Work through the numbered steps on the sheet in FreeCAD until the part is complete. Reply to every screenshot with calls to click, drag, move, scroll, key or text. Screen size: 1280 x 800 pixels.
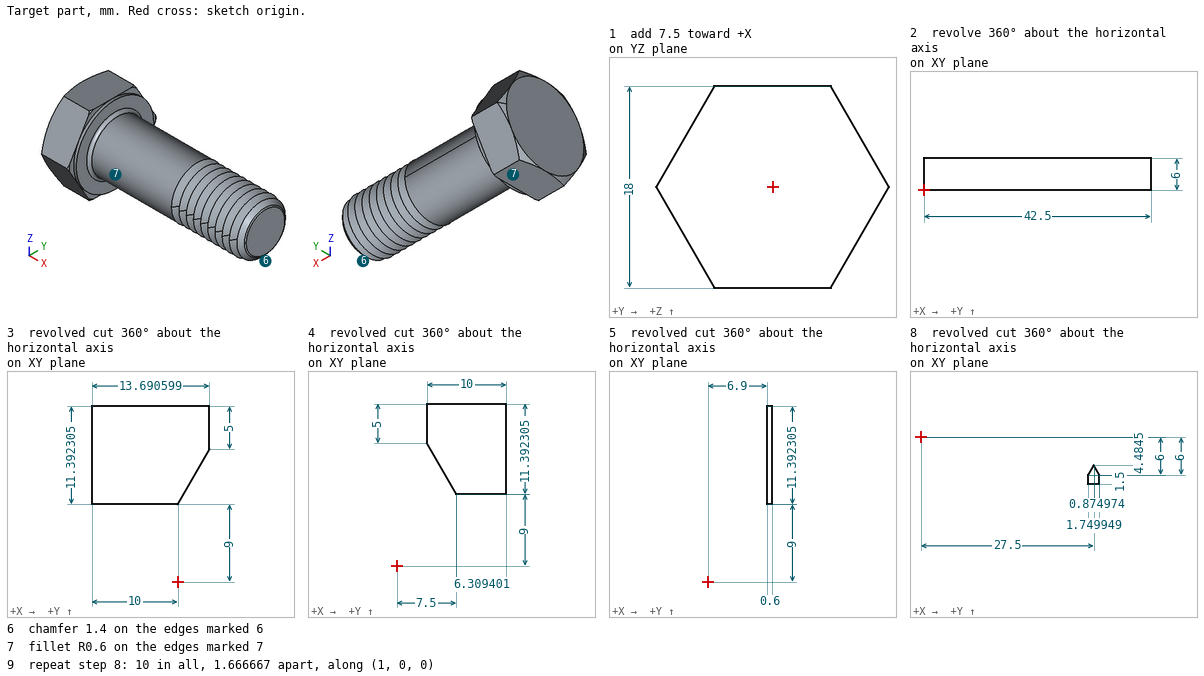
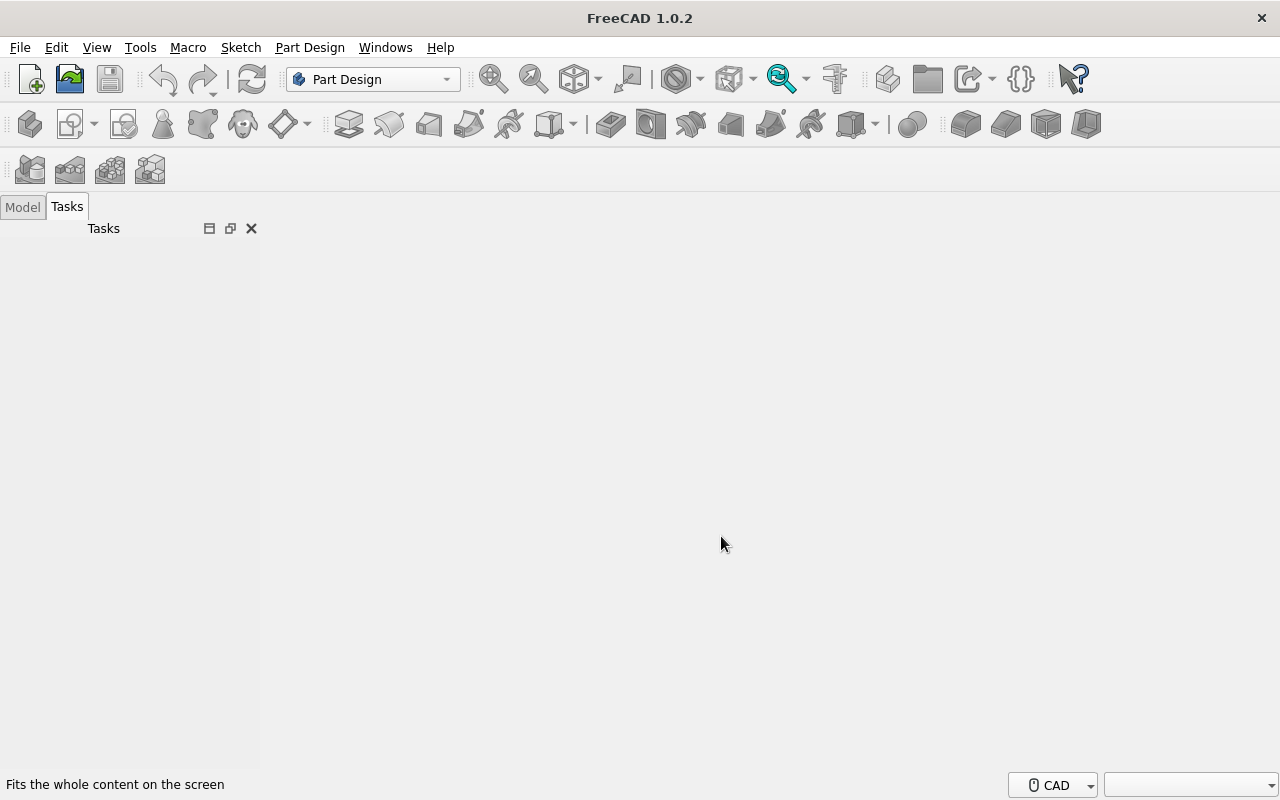
click(30, 80)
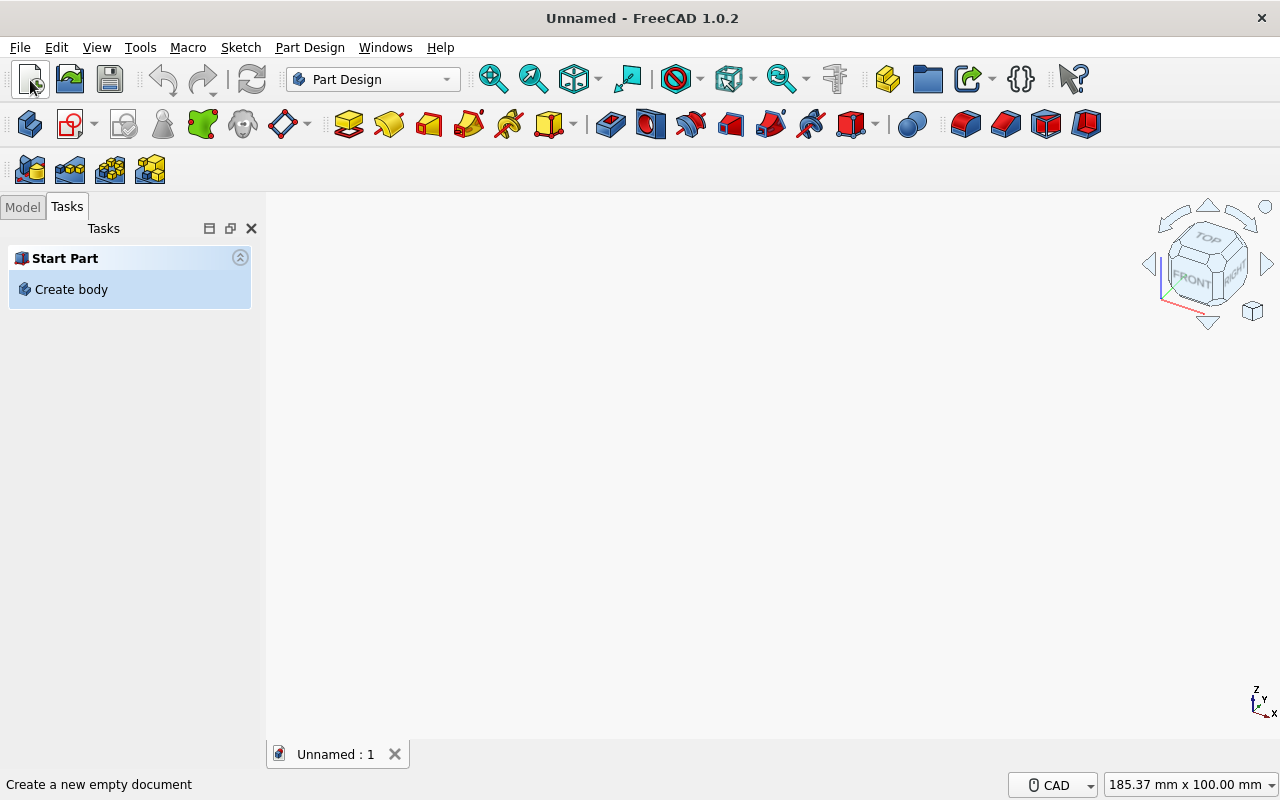
click(70, 124)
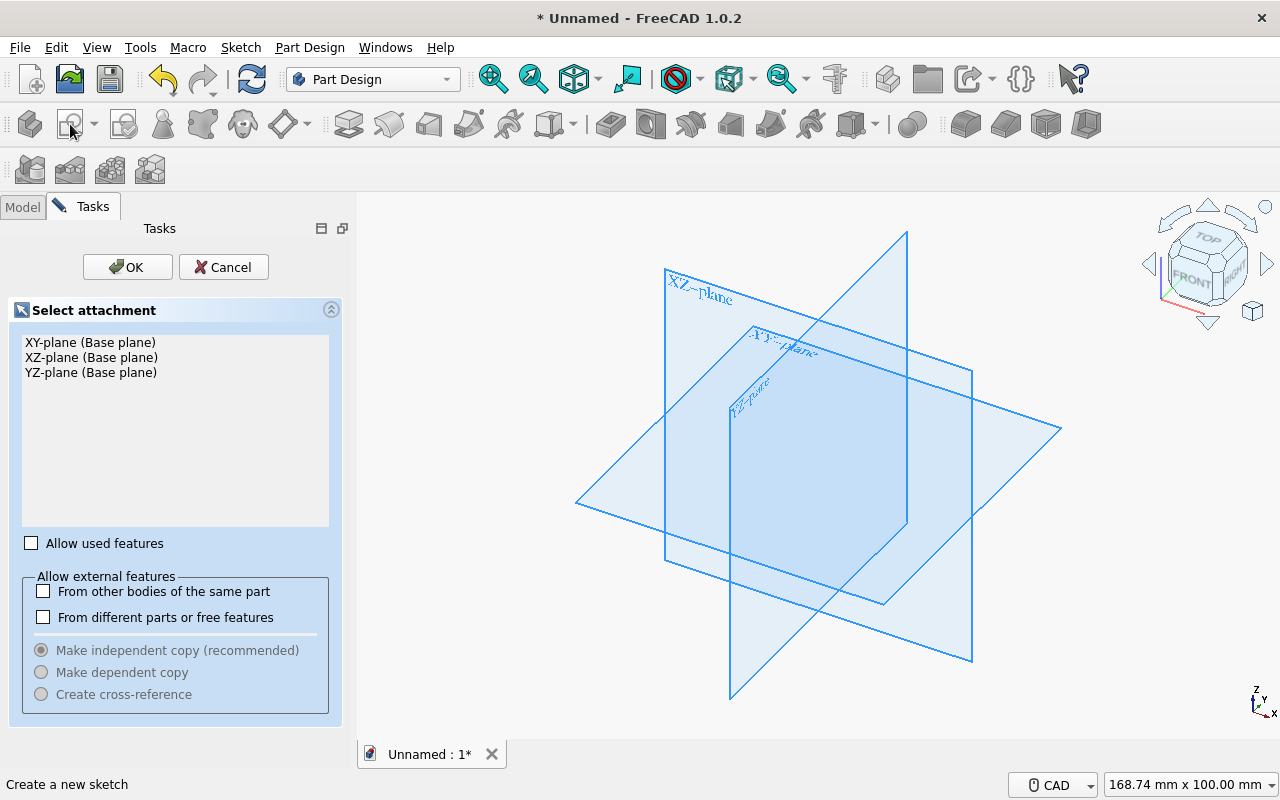
click(82, 372)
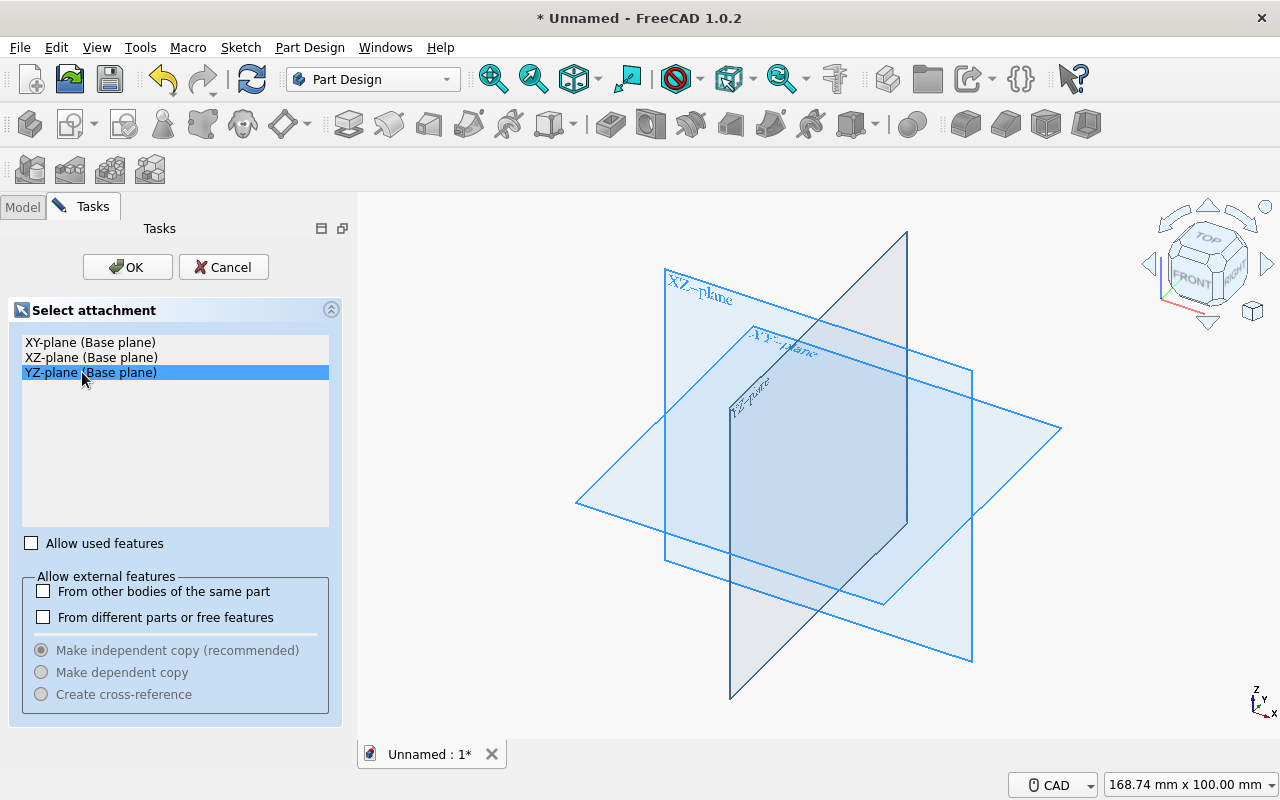
click(128, 267)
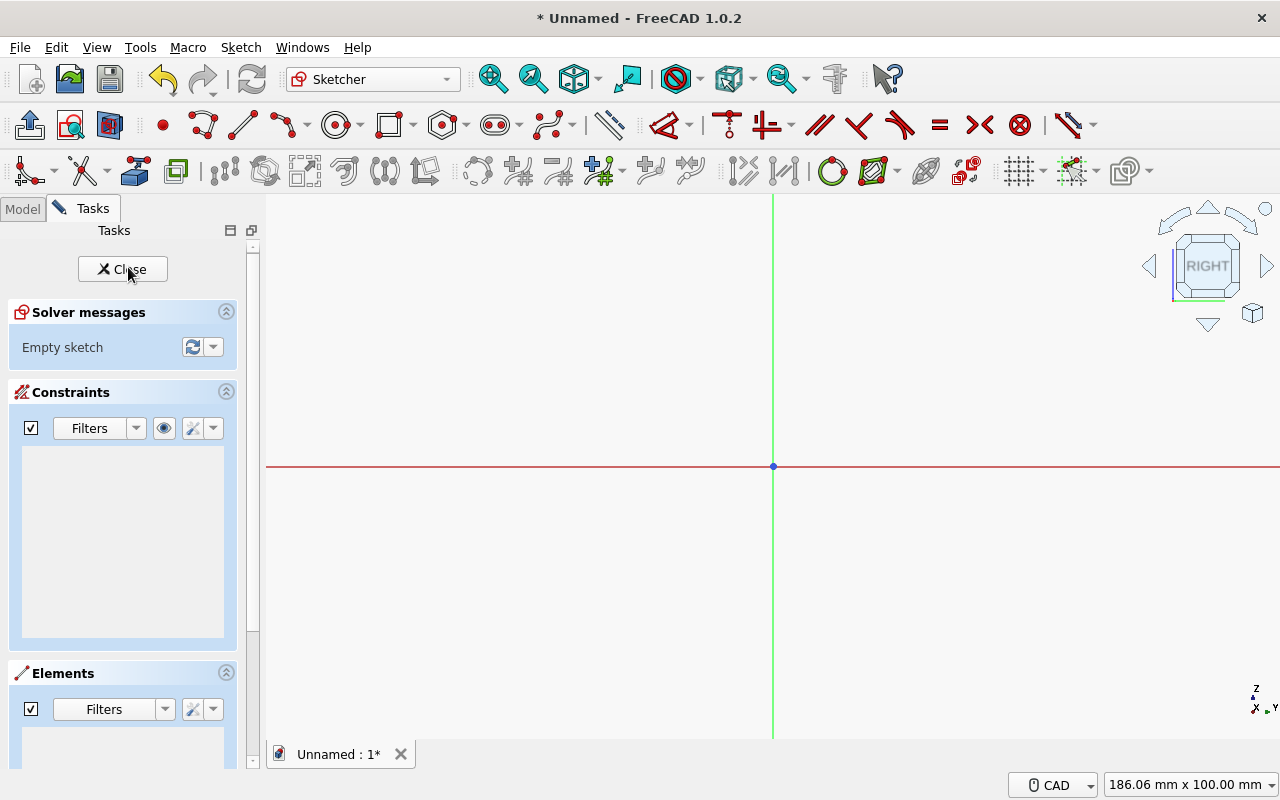
scroll(803, 466, up, 6)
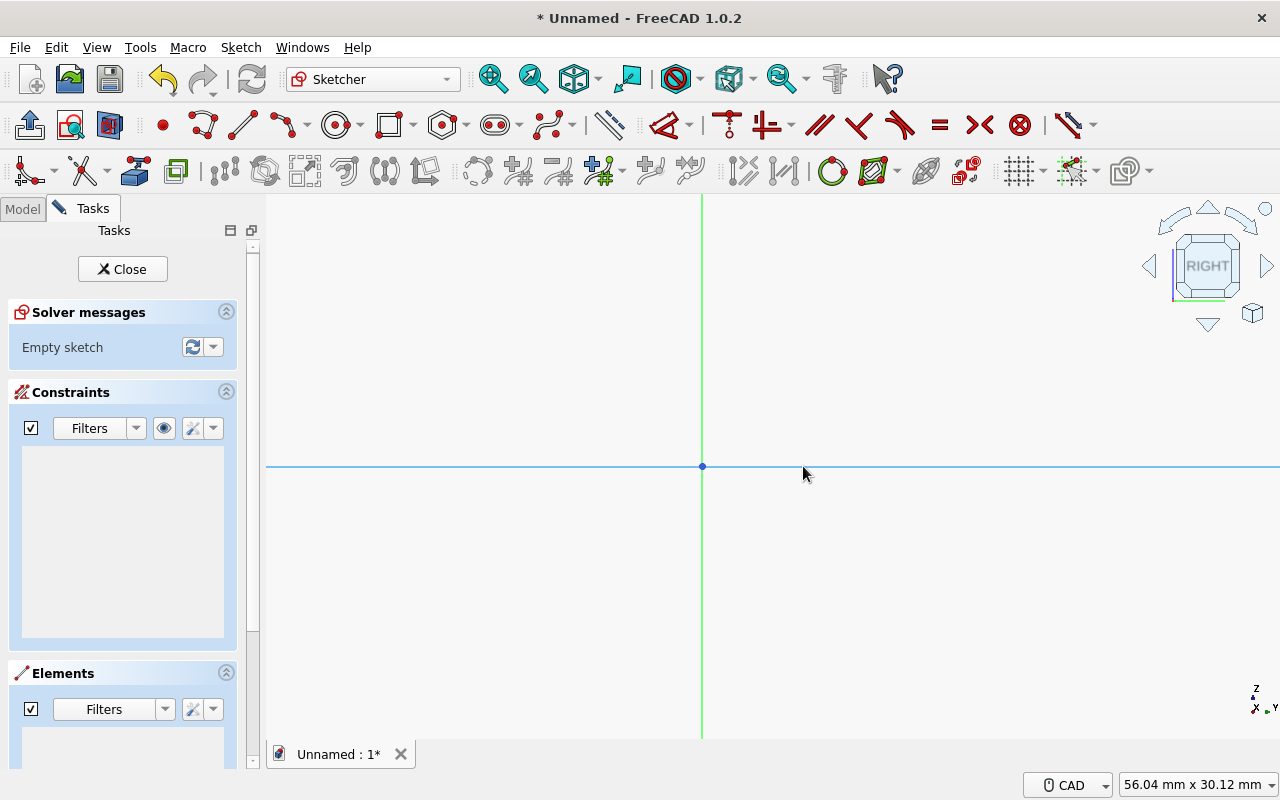
click(442, 126)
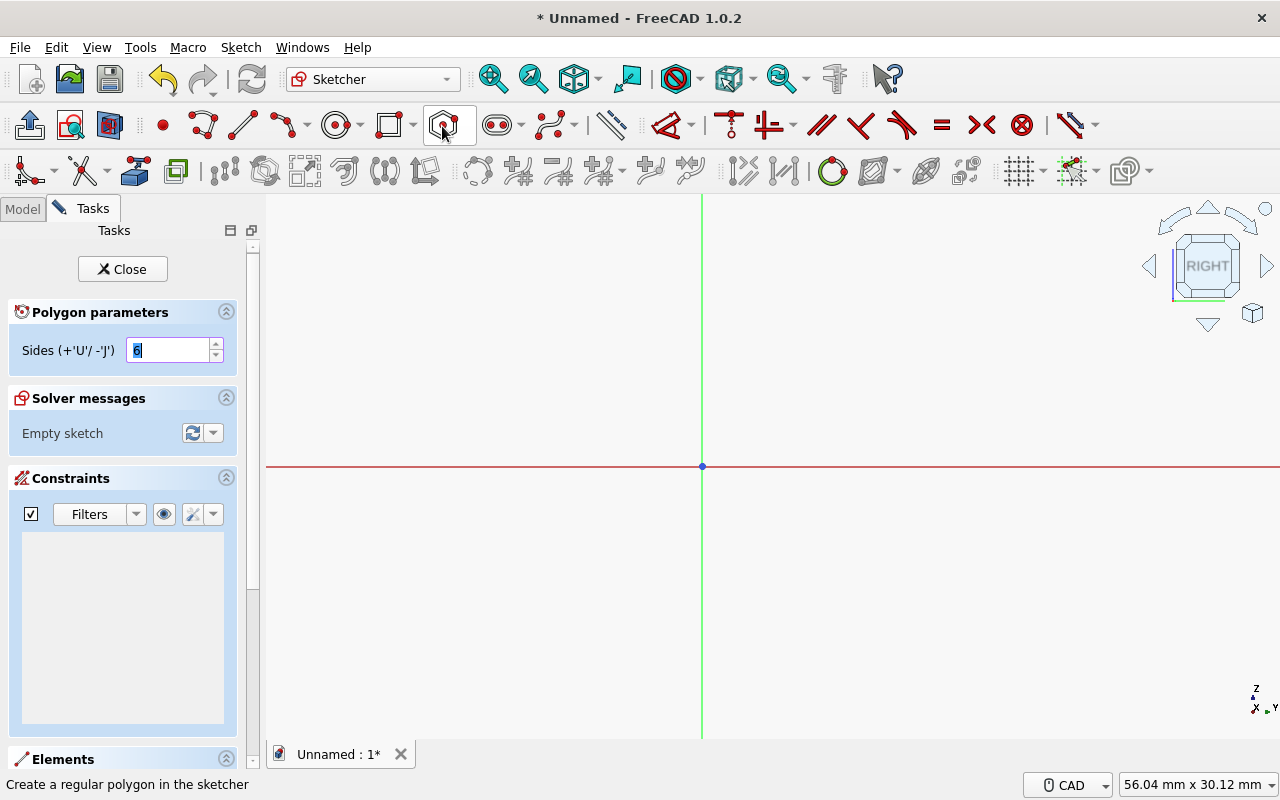
click(702, 466)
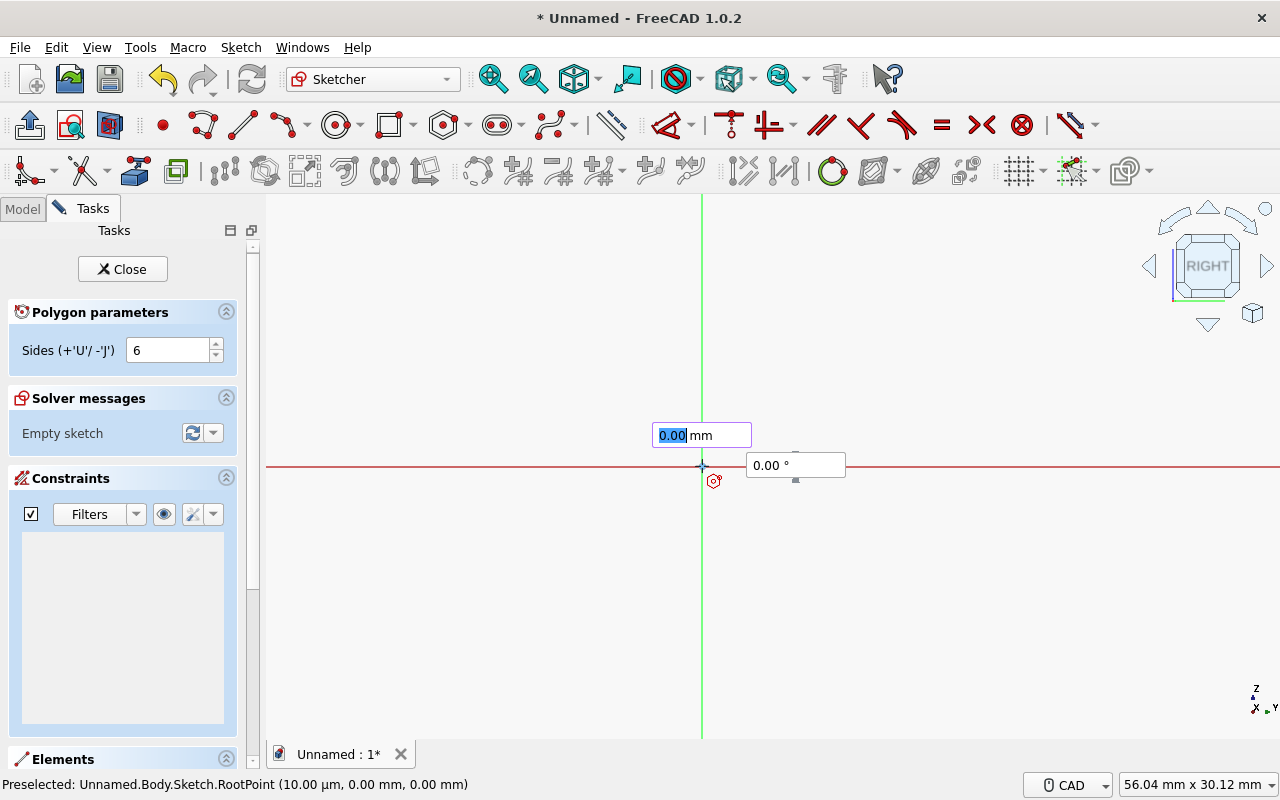
click(890, 466)
key(Escape)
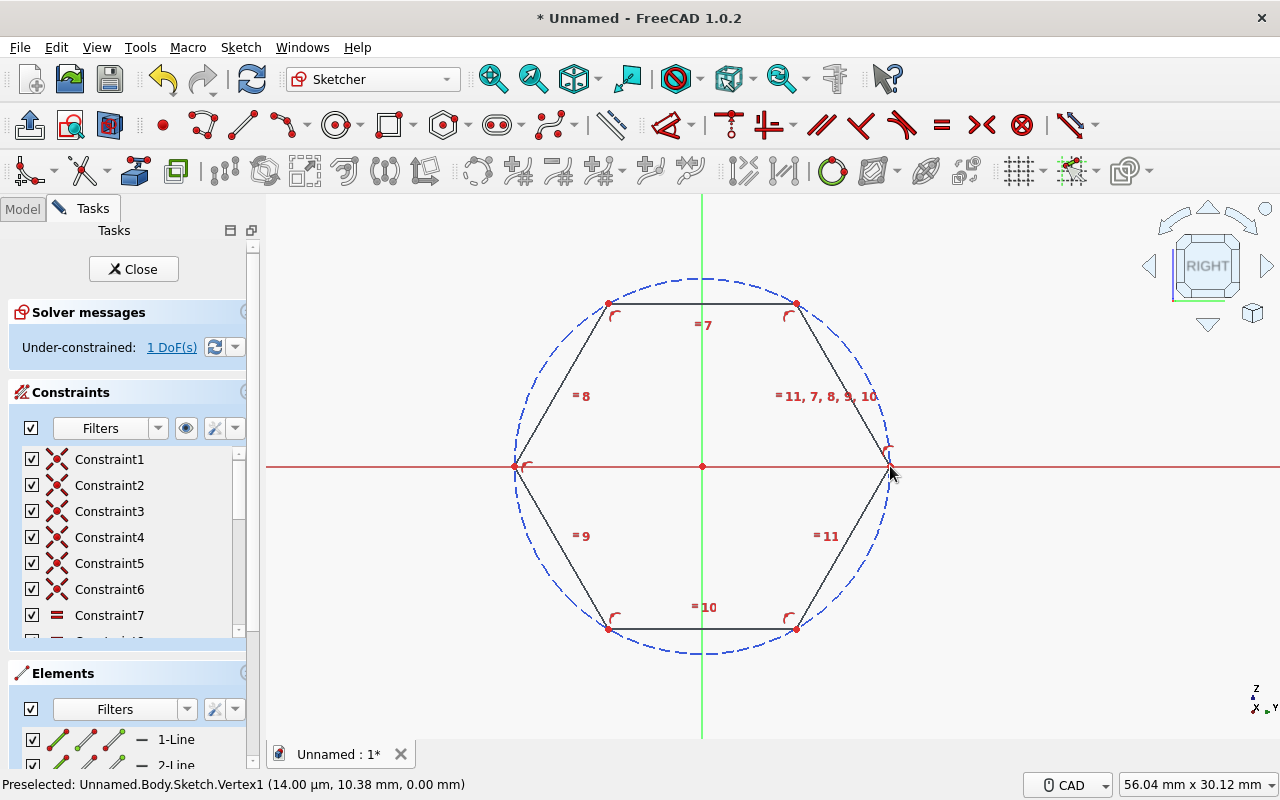
click(608, 629)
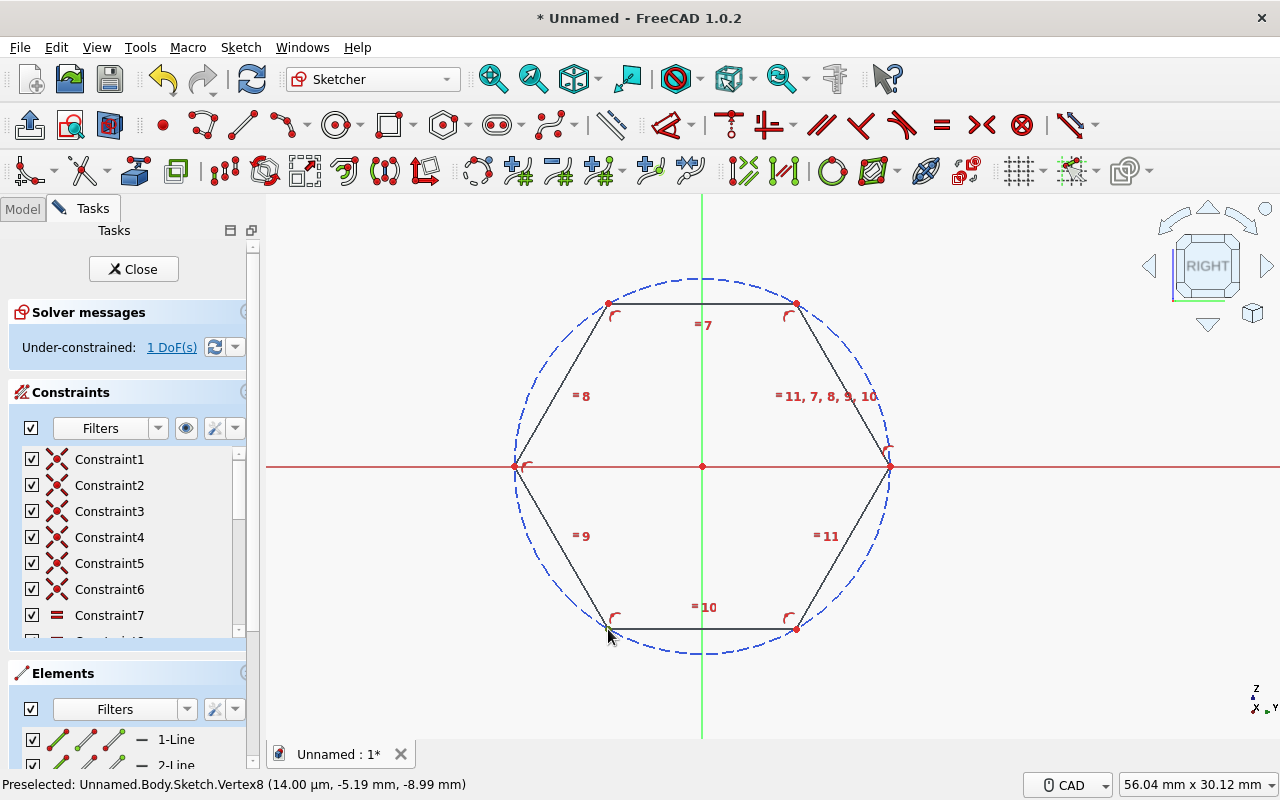
click(796, 304)